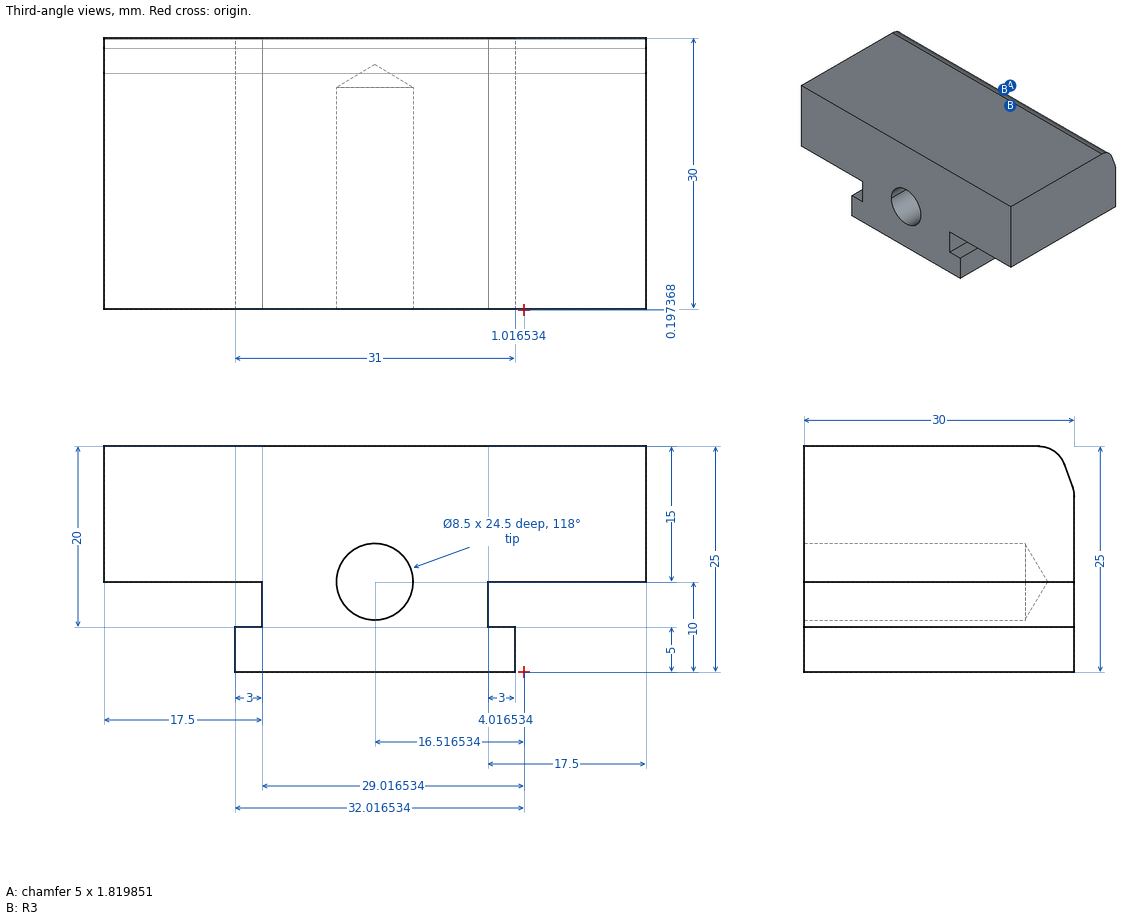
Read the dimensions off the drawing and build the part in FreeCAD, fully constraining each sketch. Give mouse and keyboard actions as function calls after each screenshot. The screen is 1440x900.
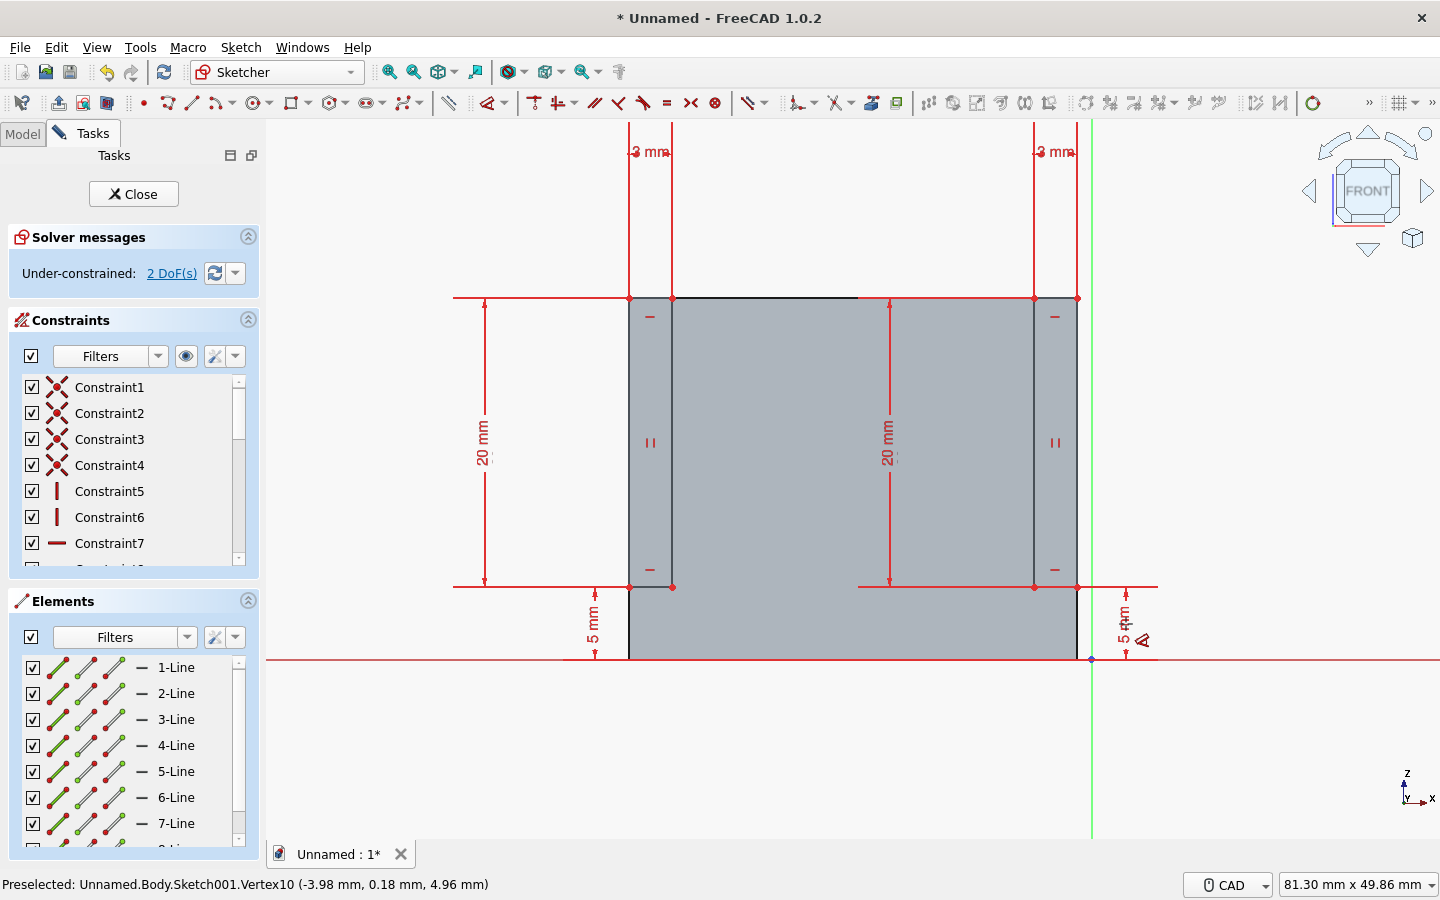
click(1034, 298)
click(1063, 694)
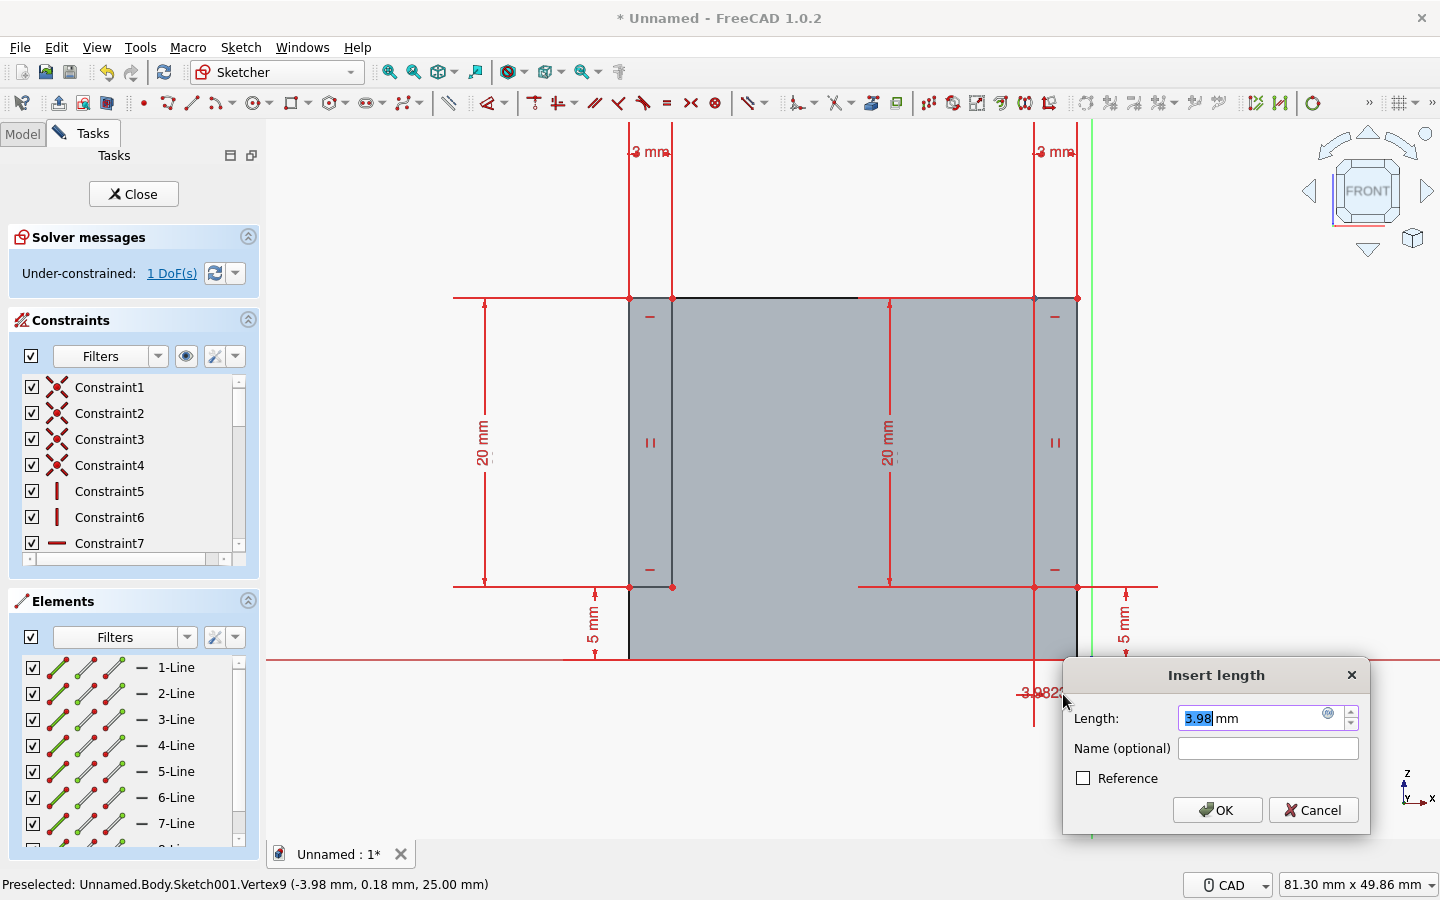
text(4.016534)
key(Return)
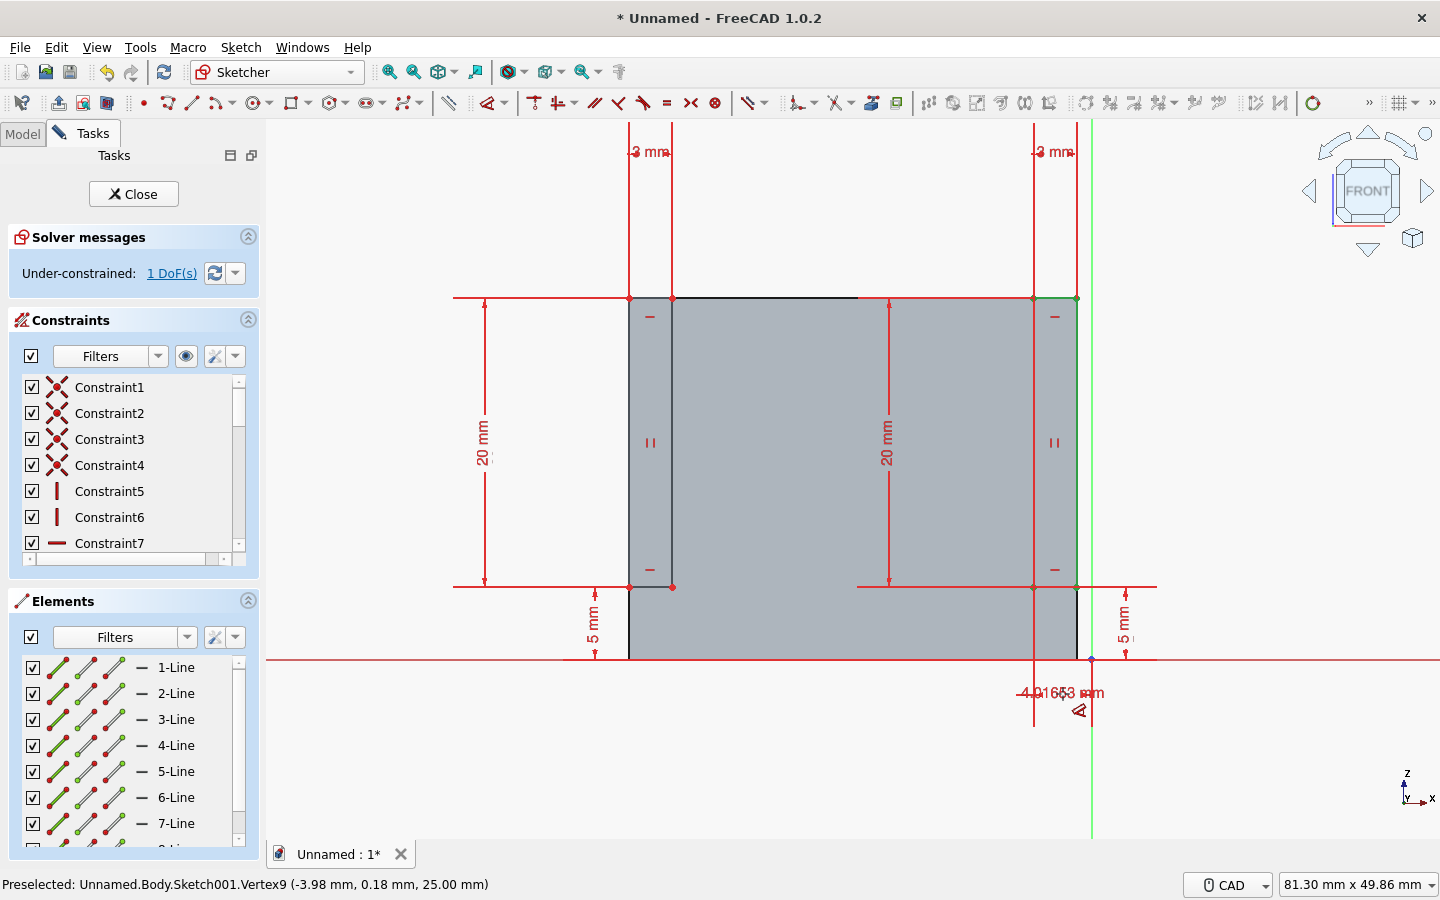
click(629, 298)
click(860, 694)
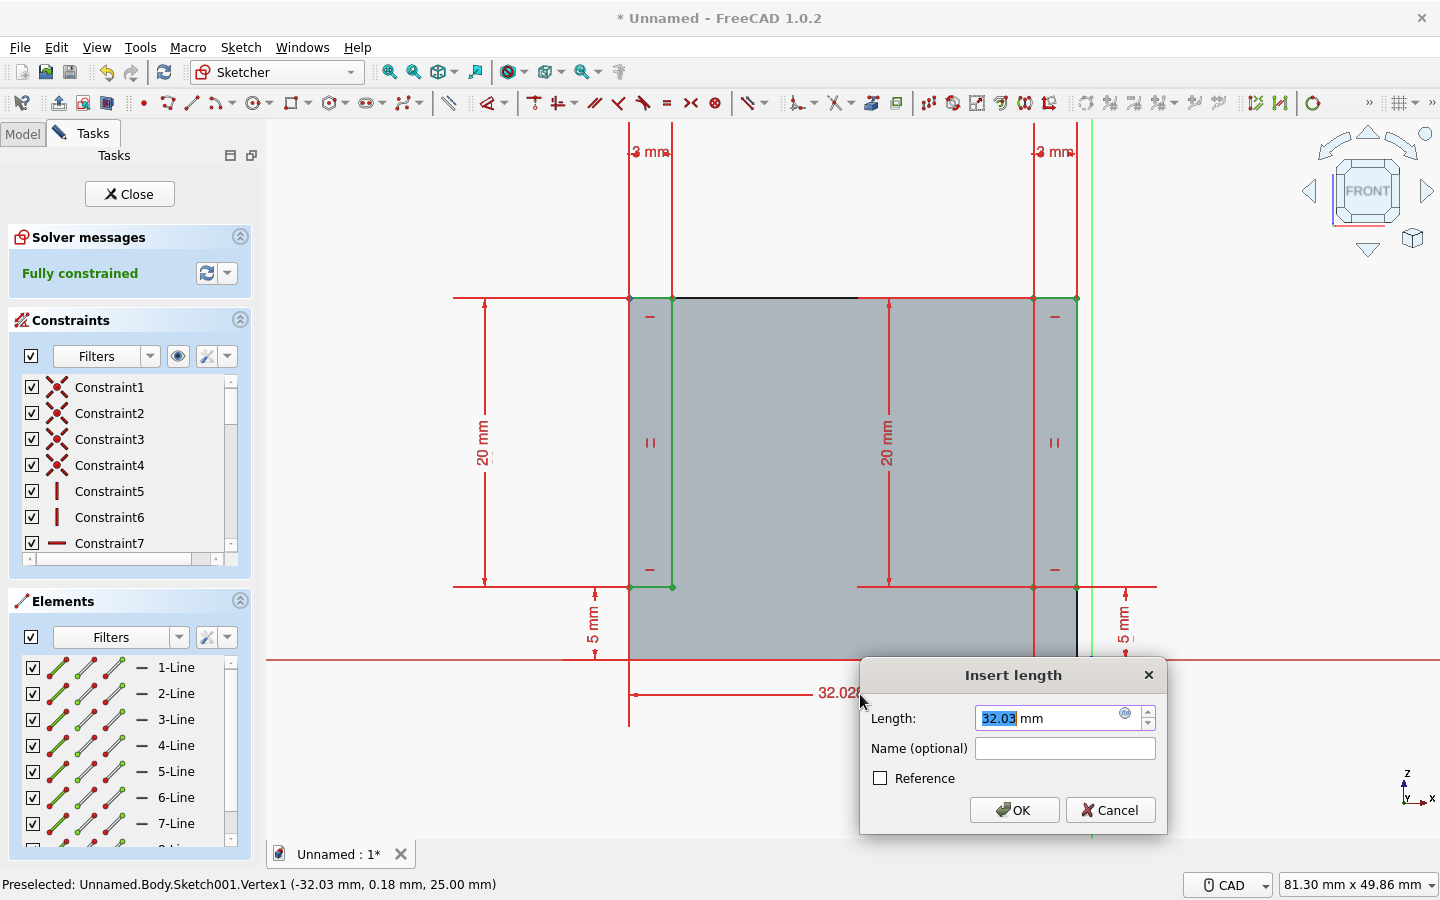
text(32.016534)
key(Return)
key(Escape)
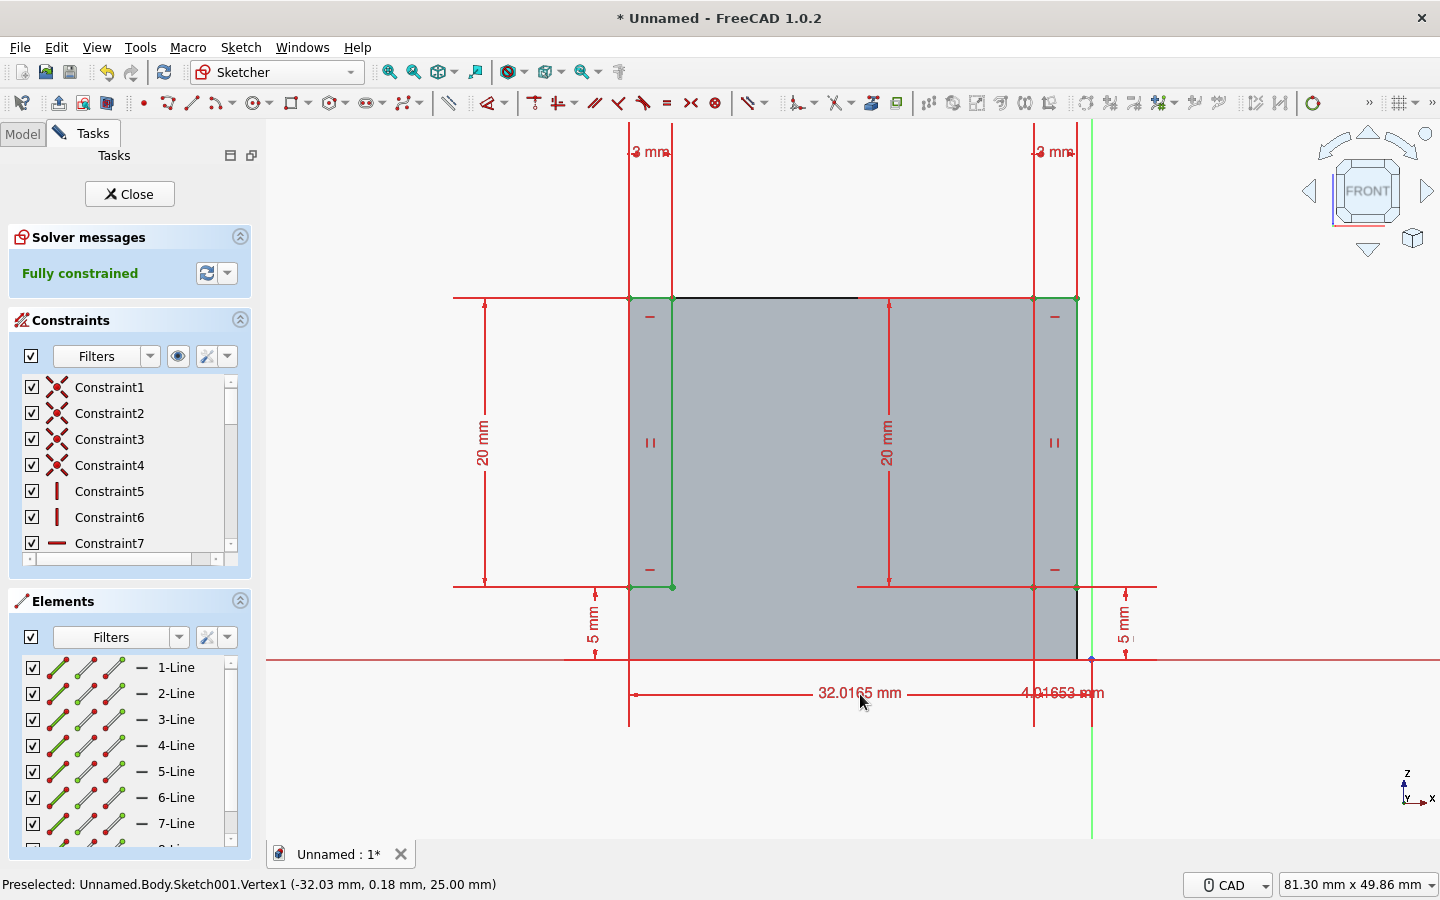
click(130, 194)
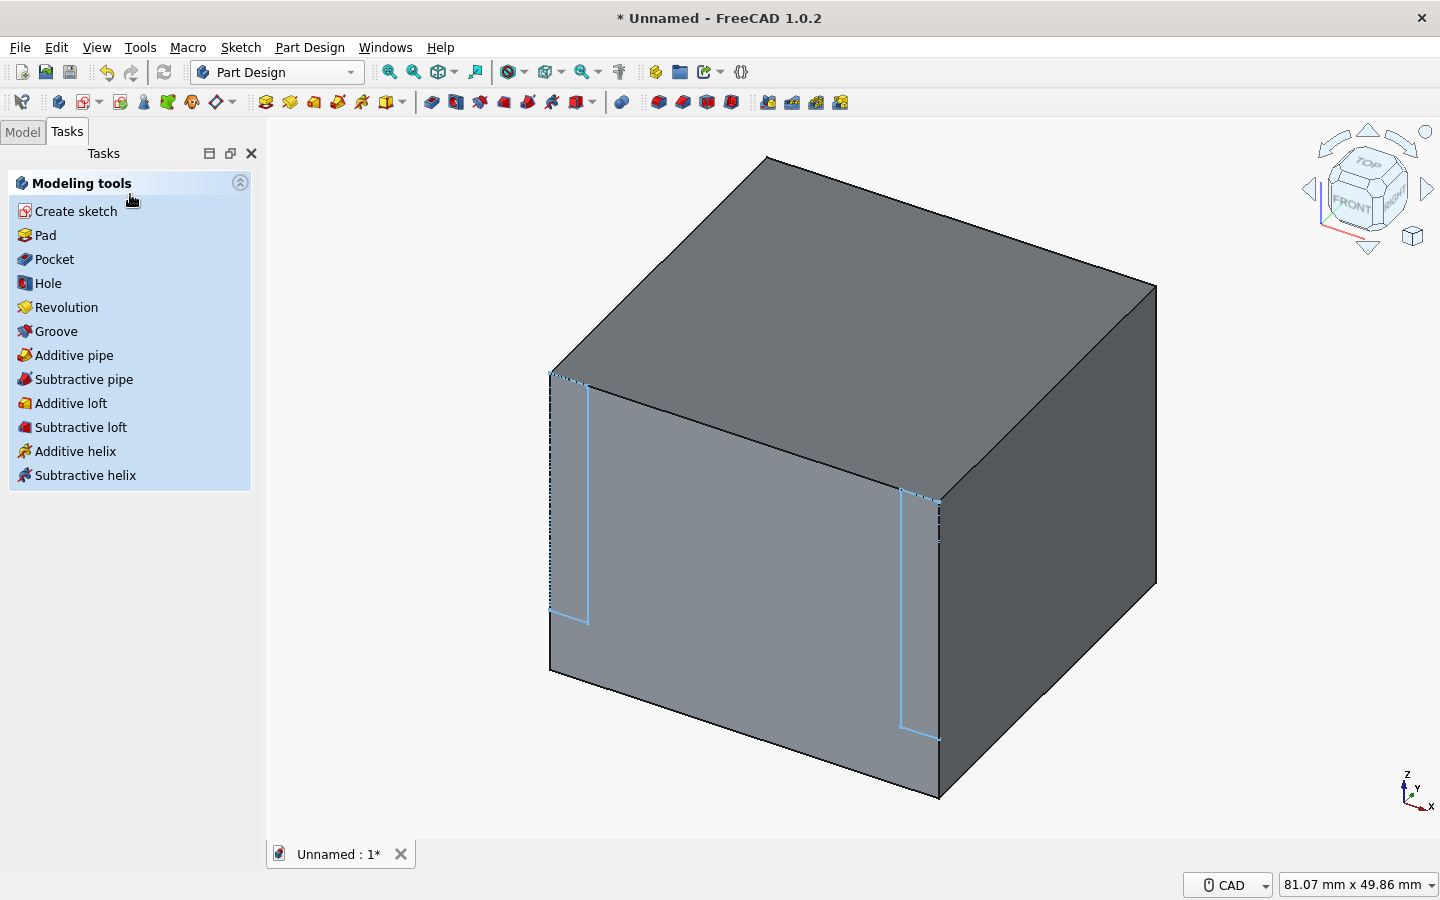
click(432, 102)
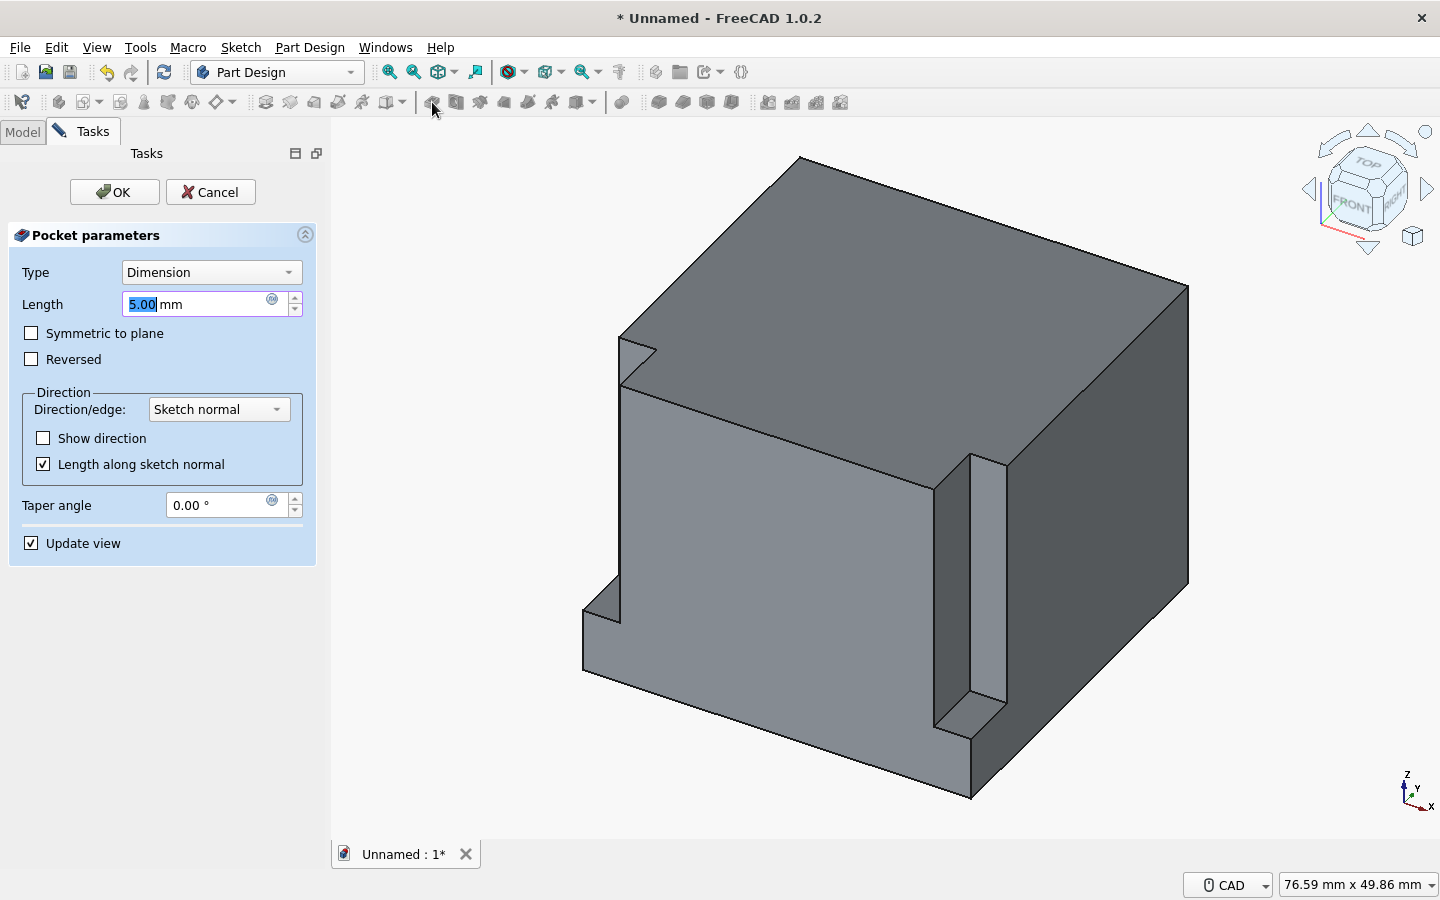
click(212, 272)